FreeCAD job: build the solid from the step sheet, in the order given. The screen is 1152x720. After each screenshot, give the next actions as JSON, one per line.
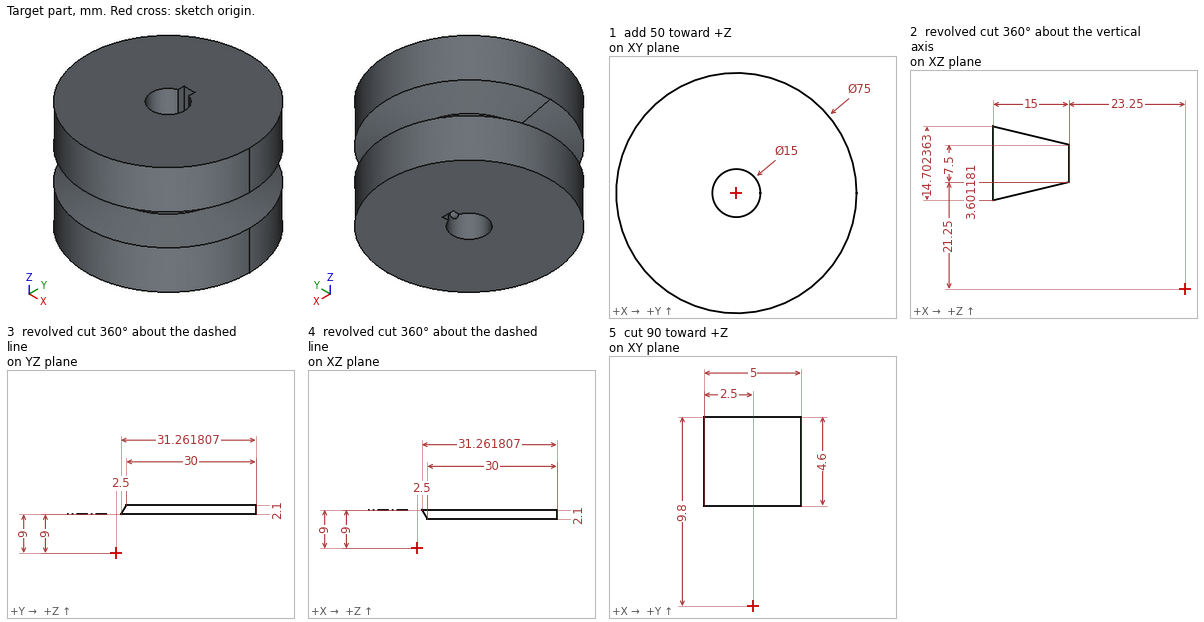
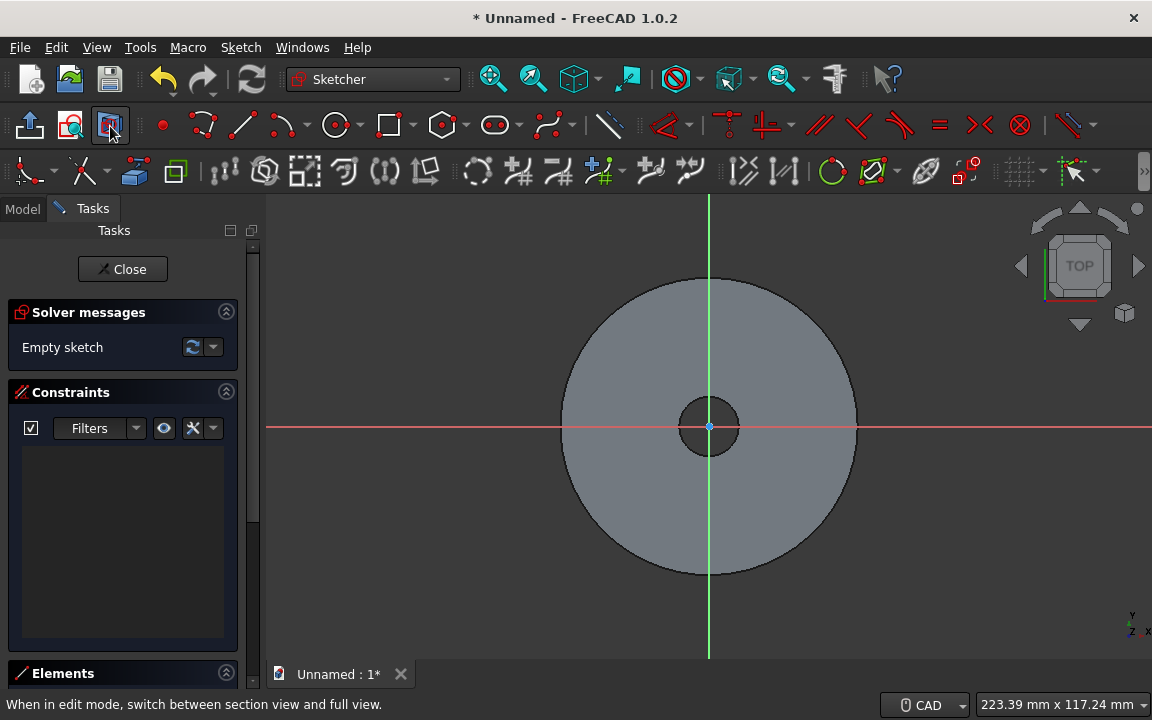
{"action": "scroll", "coordinate": [720, 404], "scroll_direction": "up", "scroll_amount": 10}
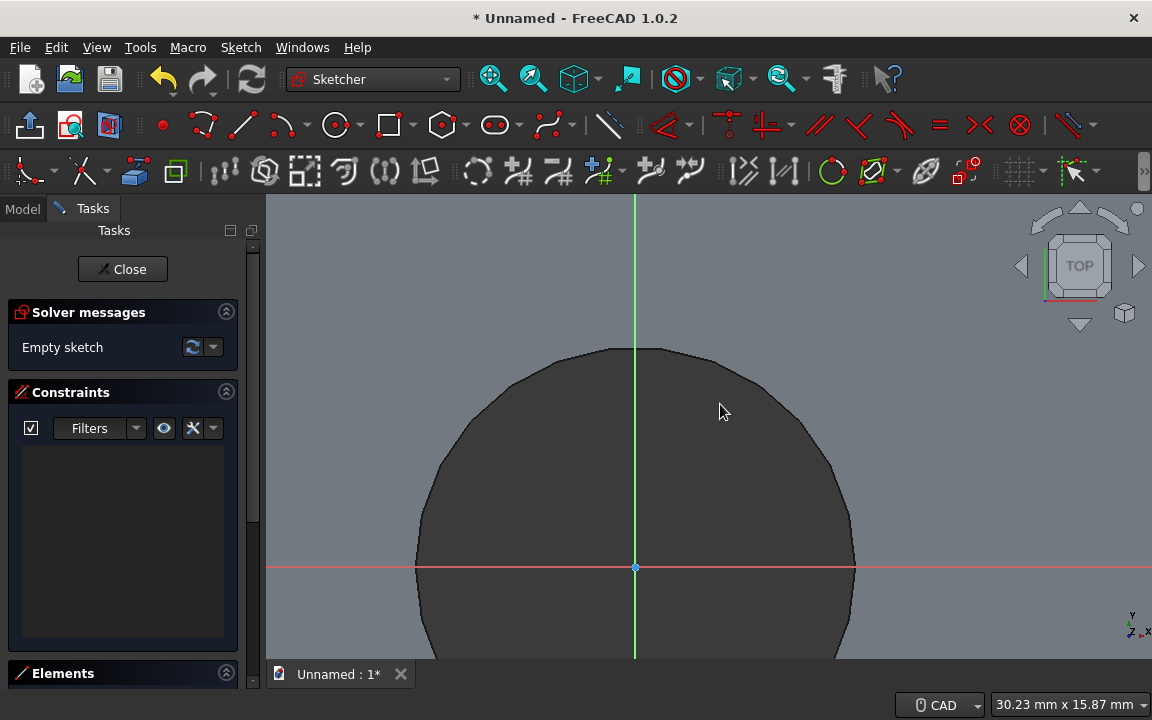
{"action": "left_click", "coordinate": [390, 126]}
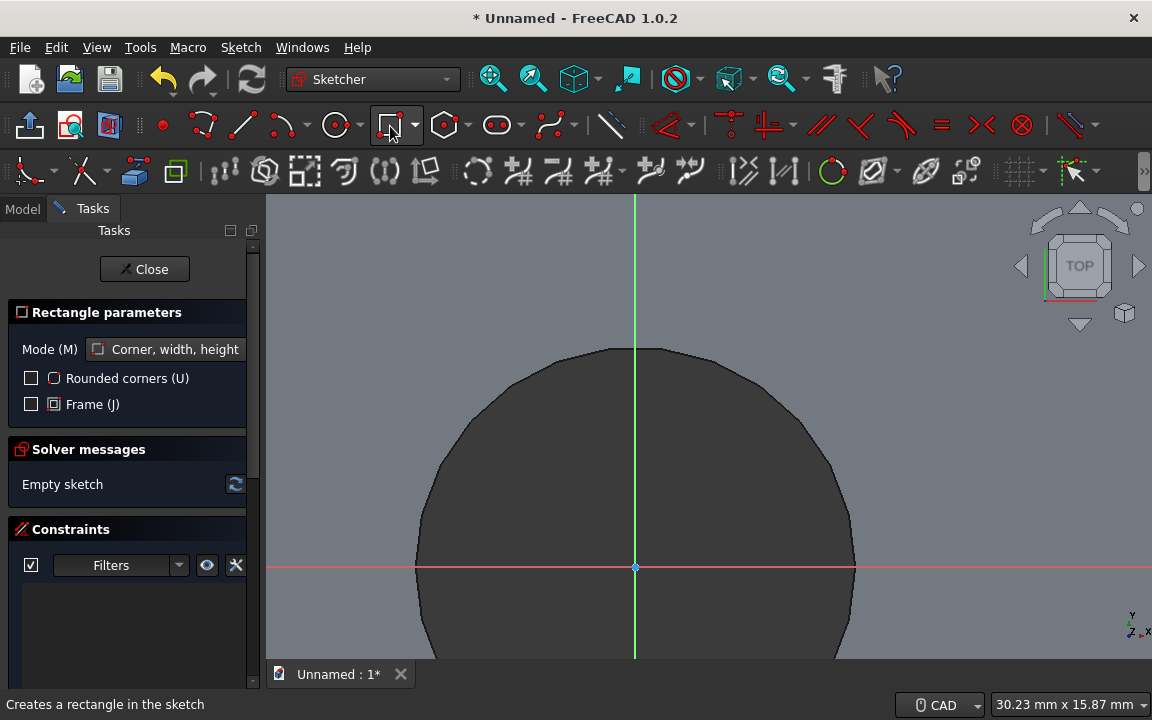
{"action": "left_click", "coordinate": [562, 280]}
{"action": "mouse_move", "coordinate": [709, 415]}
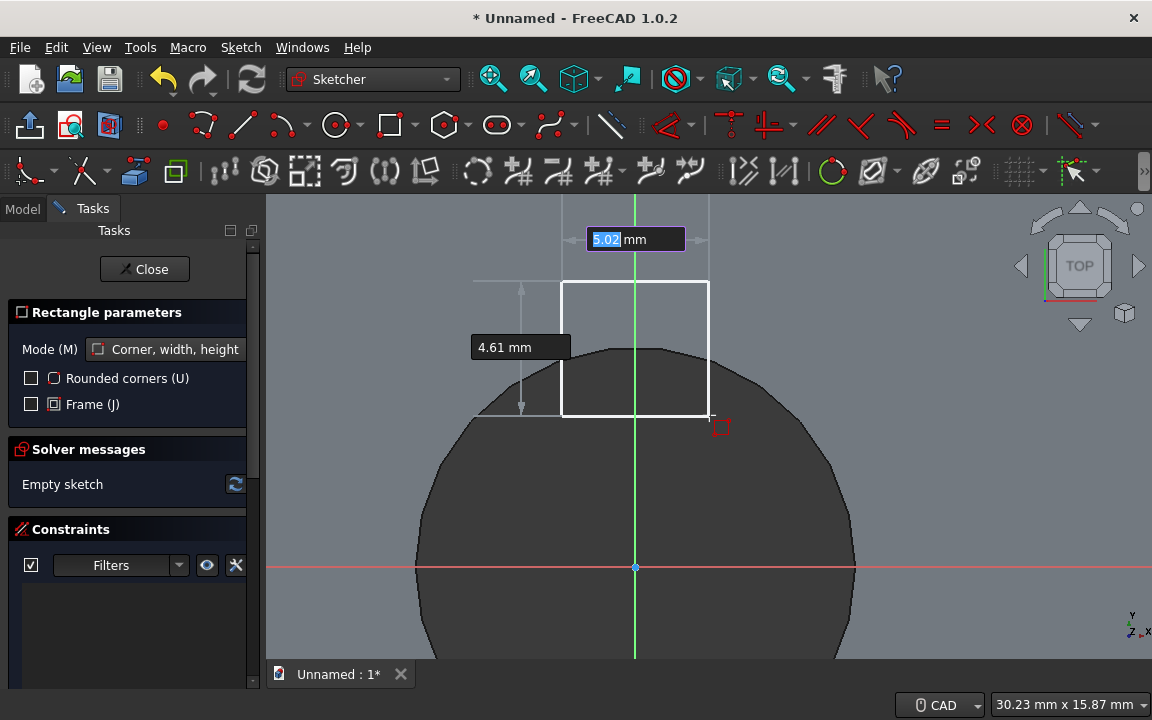
{"action": "type", "text": "5"}
{"action": "key", "text": "Tab"}
{"action": "type", "text": "4.6"}
{"action": "key", "text": "Return"}
{"action": "key", "text": "Escape"}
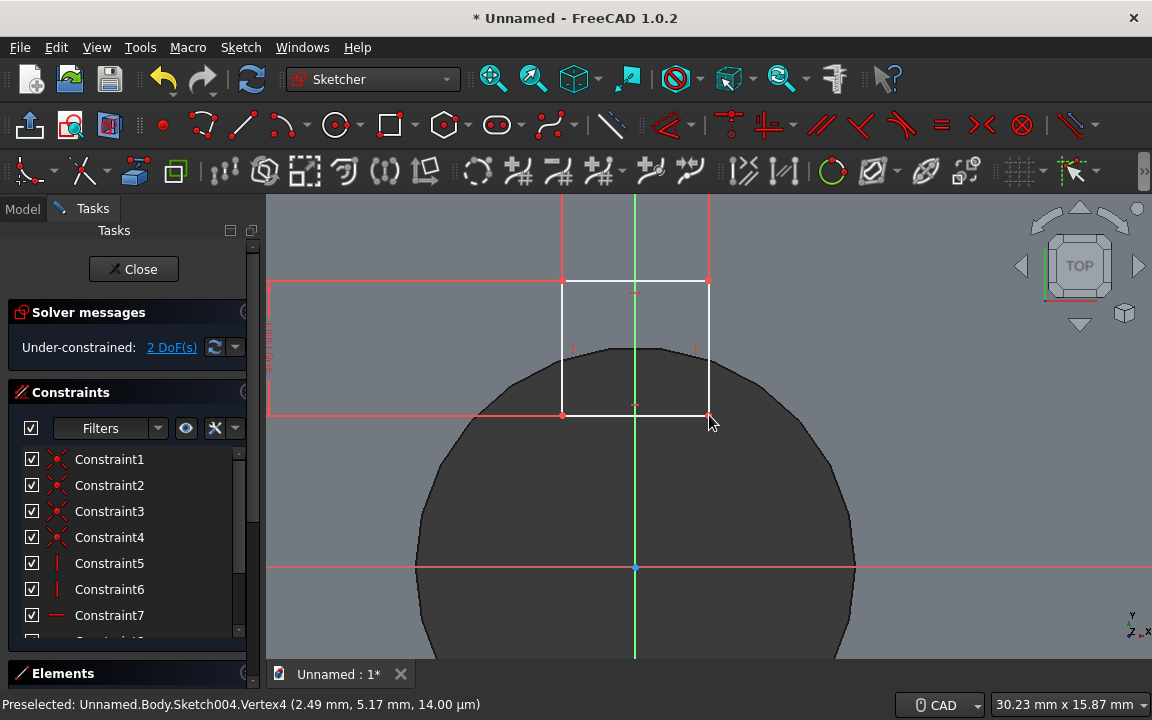
{"action": "key", "text": "d"}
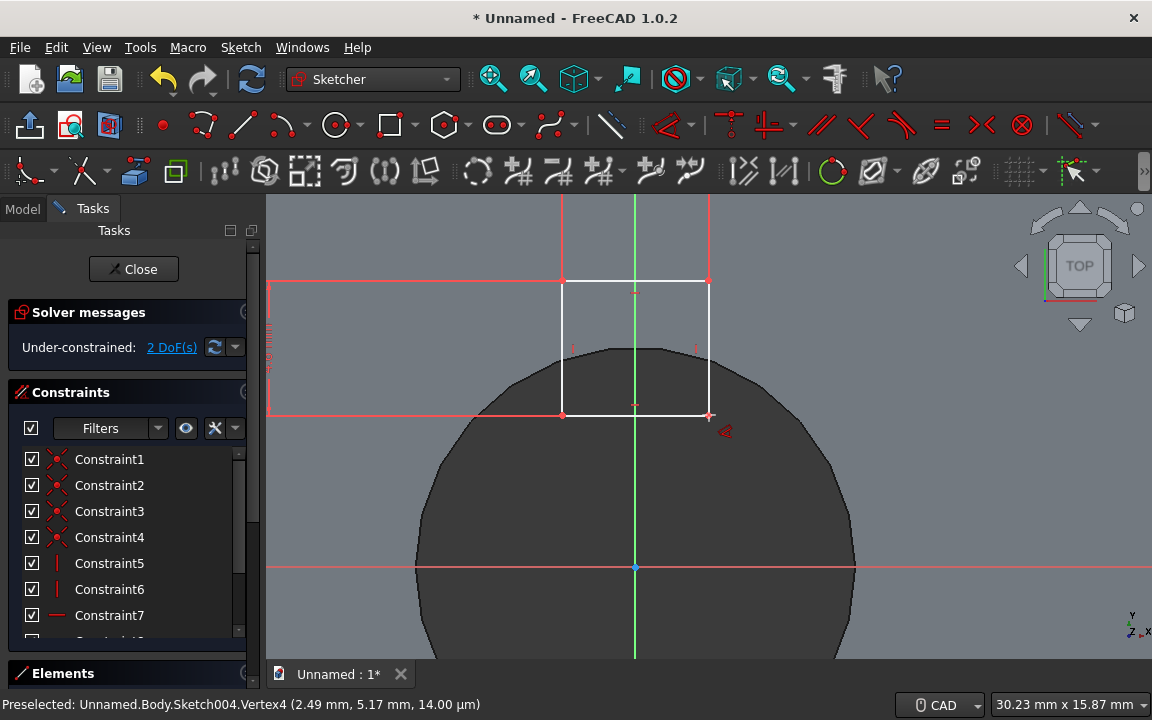
{"action": "left_click", "coordinate": [562, 281]}
{"action": "left_click", "coordinate": [599, 601]}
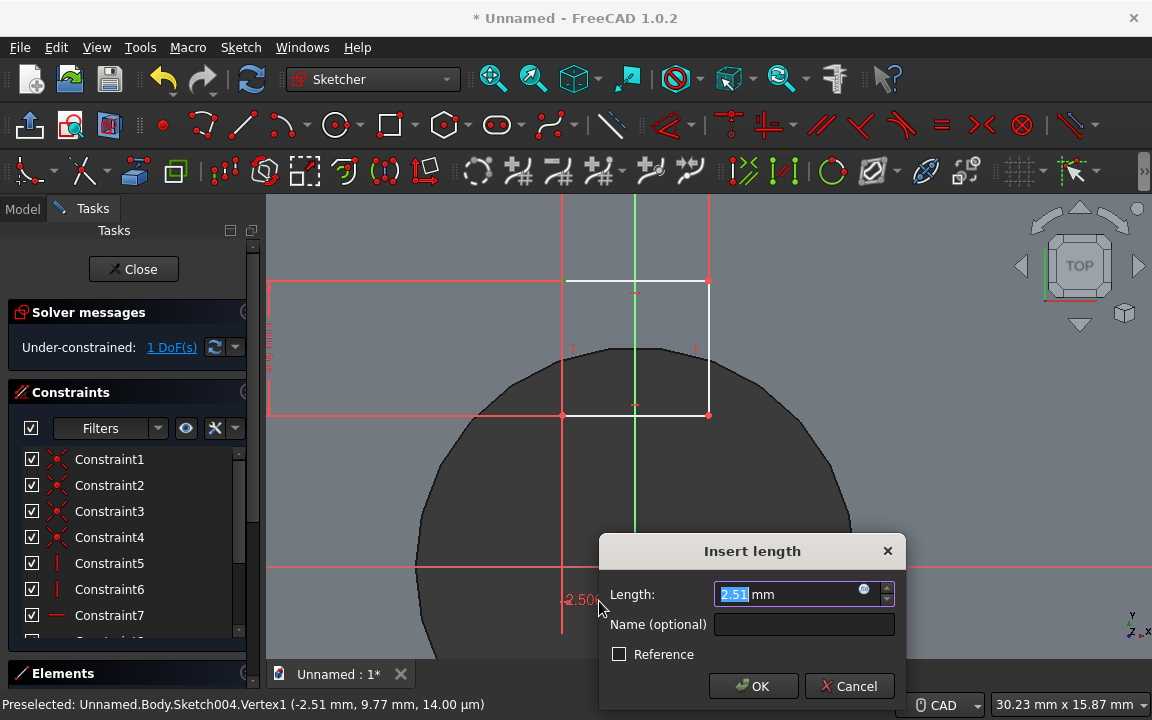
{"action": "type", "text": "2.5"}
{"action": "key", "text": "Return"}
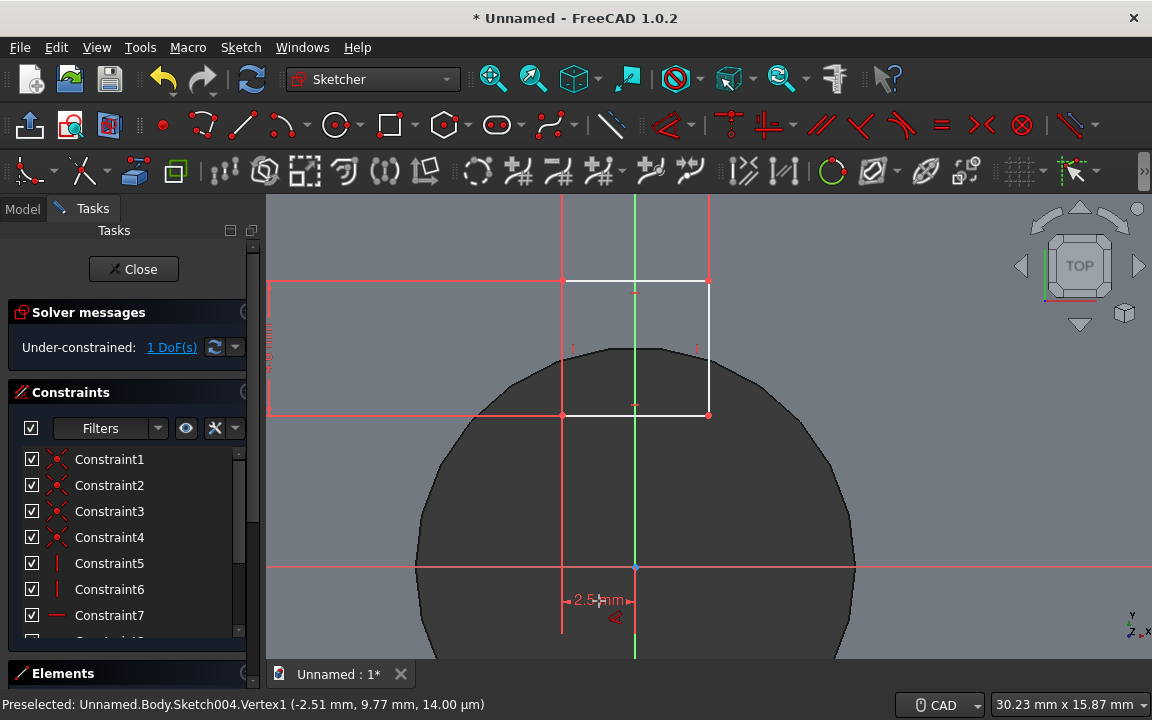
{"action": "left_click", "coordinate": [562, 281]}
{"action": "left_click", "coordinate": [528, 424]}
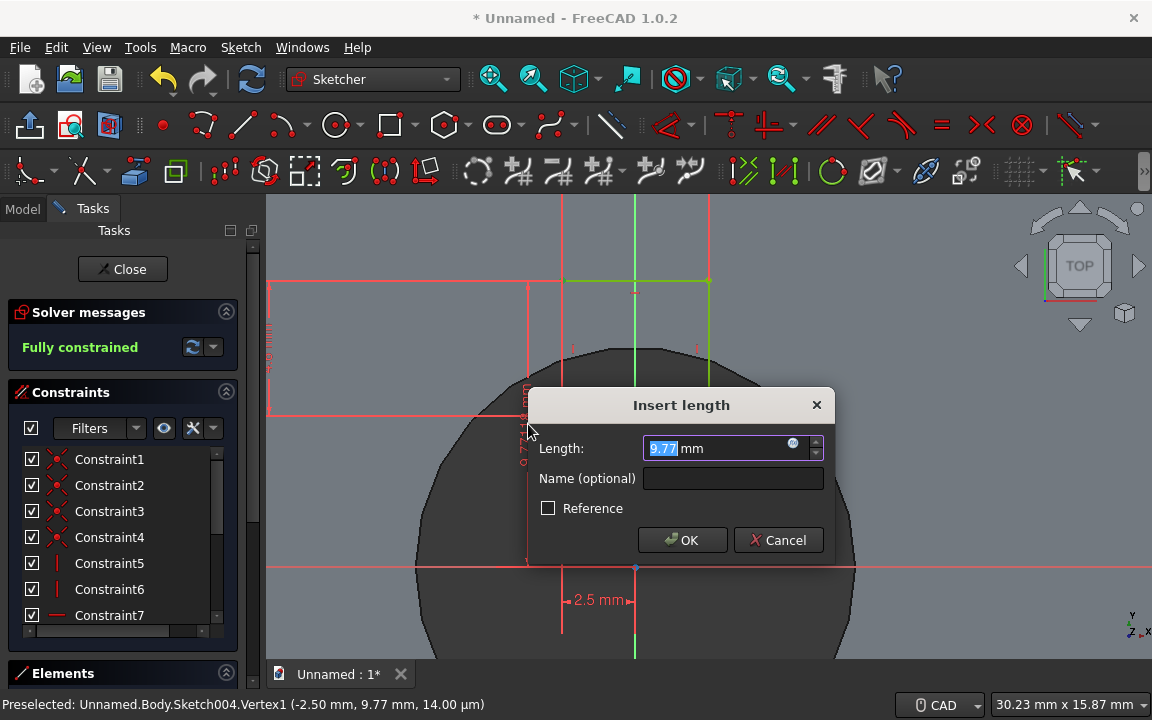
{"action": "type", "text": "9.8"}
{"action": "key", "text": "Return"}
{"action": "key", "text": "Escape"}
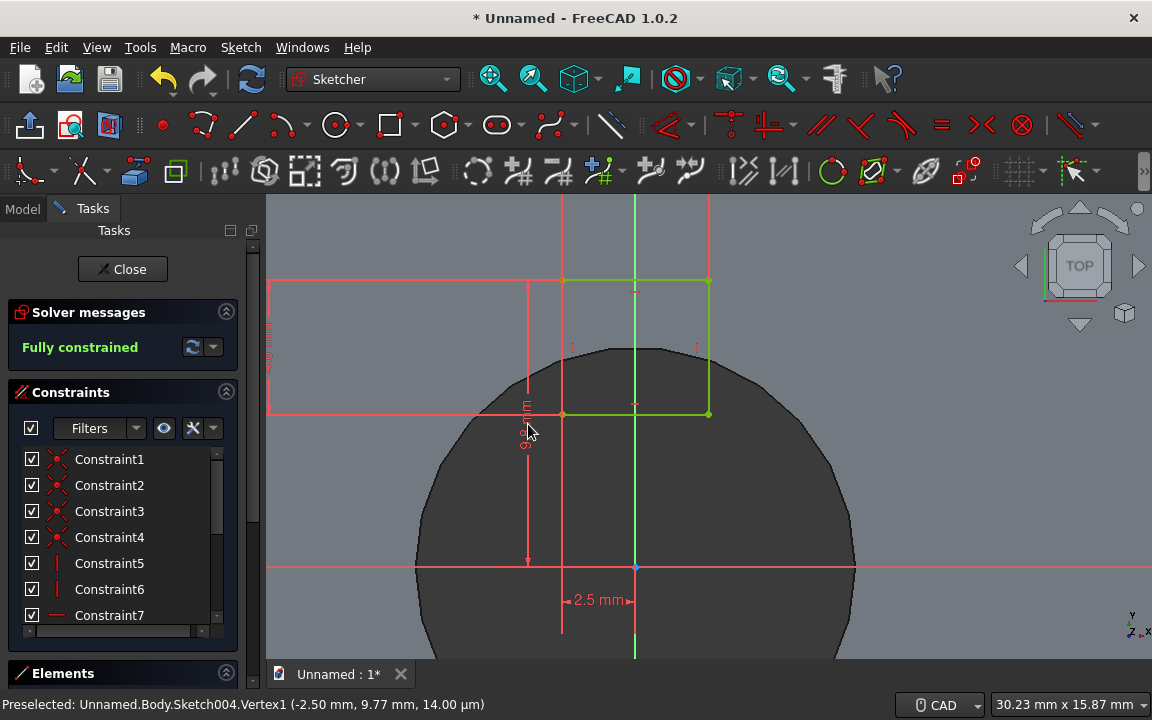
{"action": "left_click", "coordinate": [123, 269]}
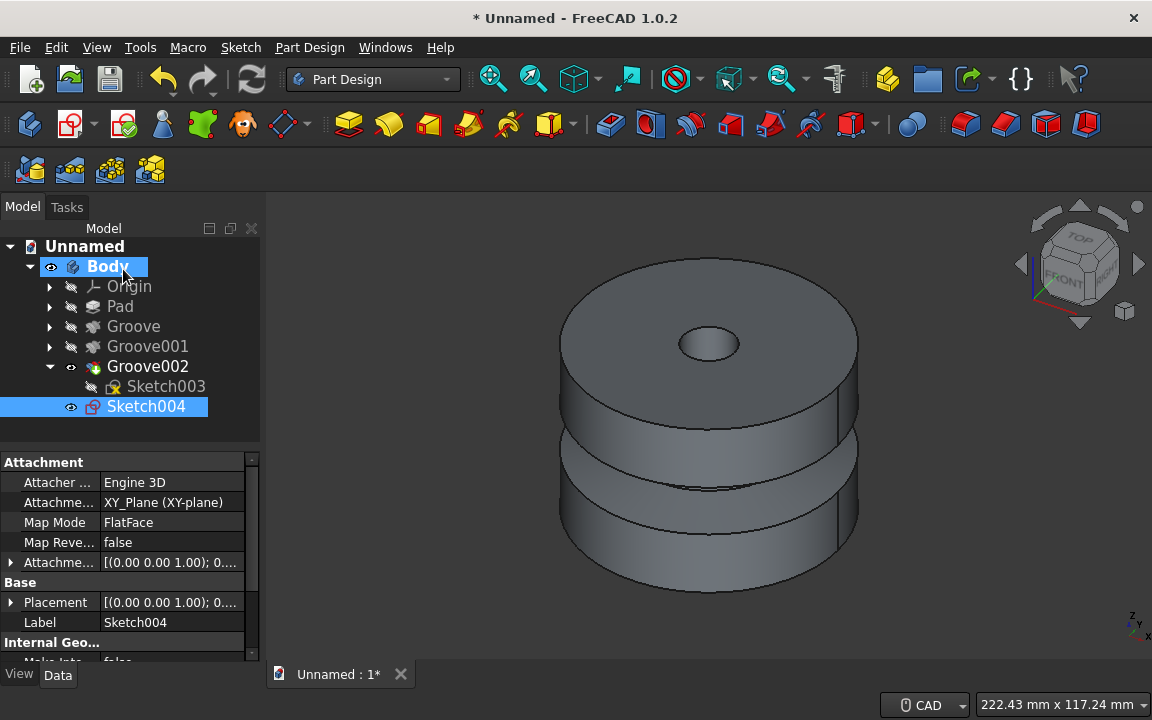
{"action": "left_click", "coordinate": [612, 124]}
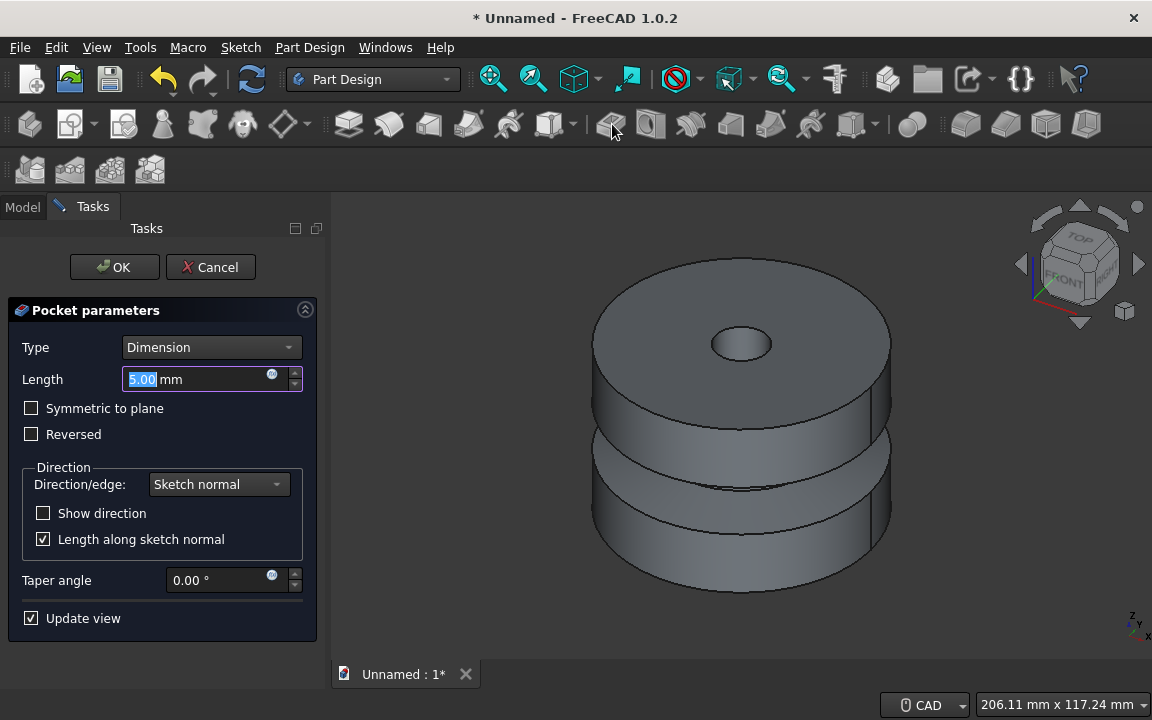
{"action": "type", "text": "90"}
{"action": "key", "text": "Tab"}